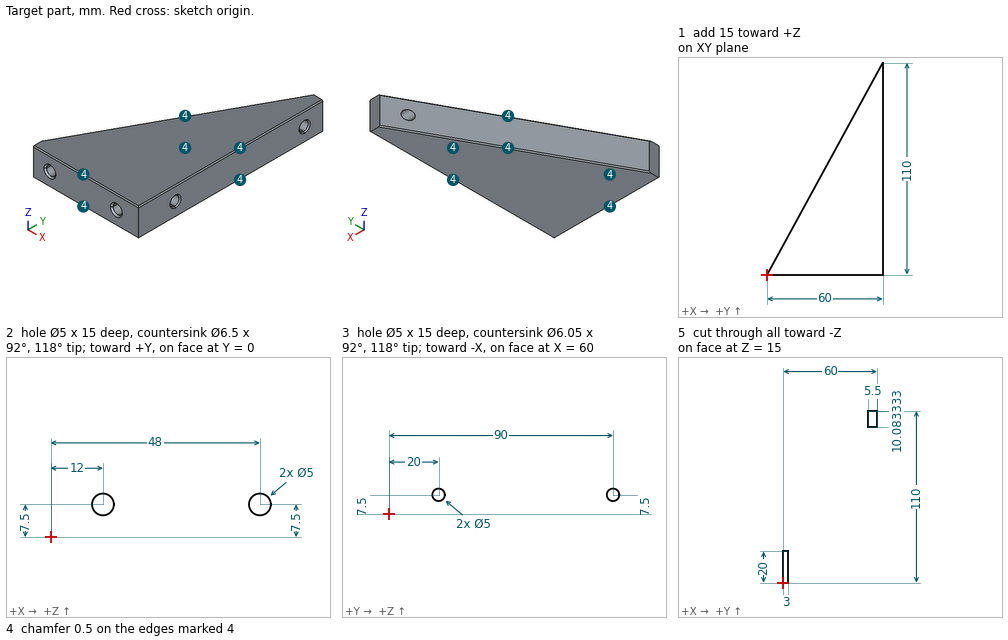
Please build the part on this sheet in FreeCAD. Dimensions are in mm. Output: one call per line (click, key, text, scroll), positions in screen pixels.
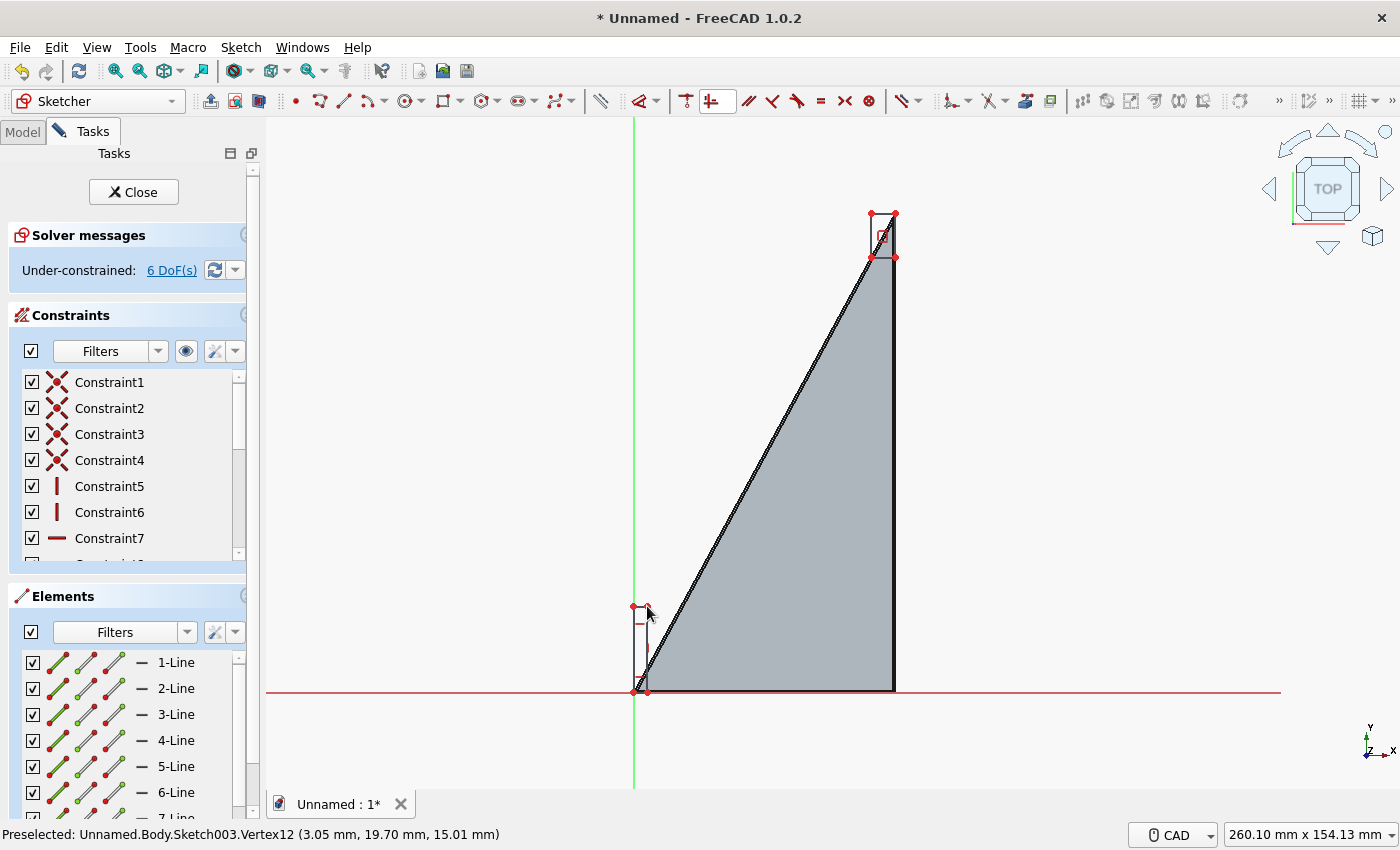
click(640, 102)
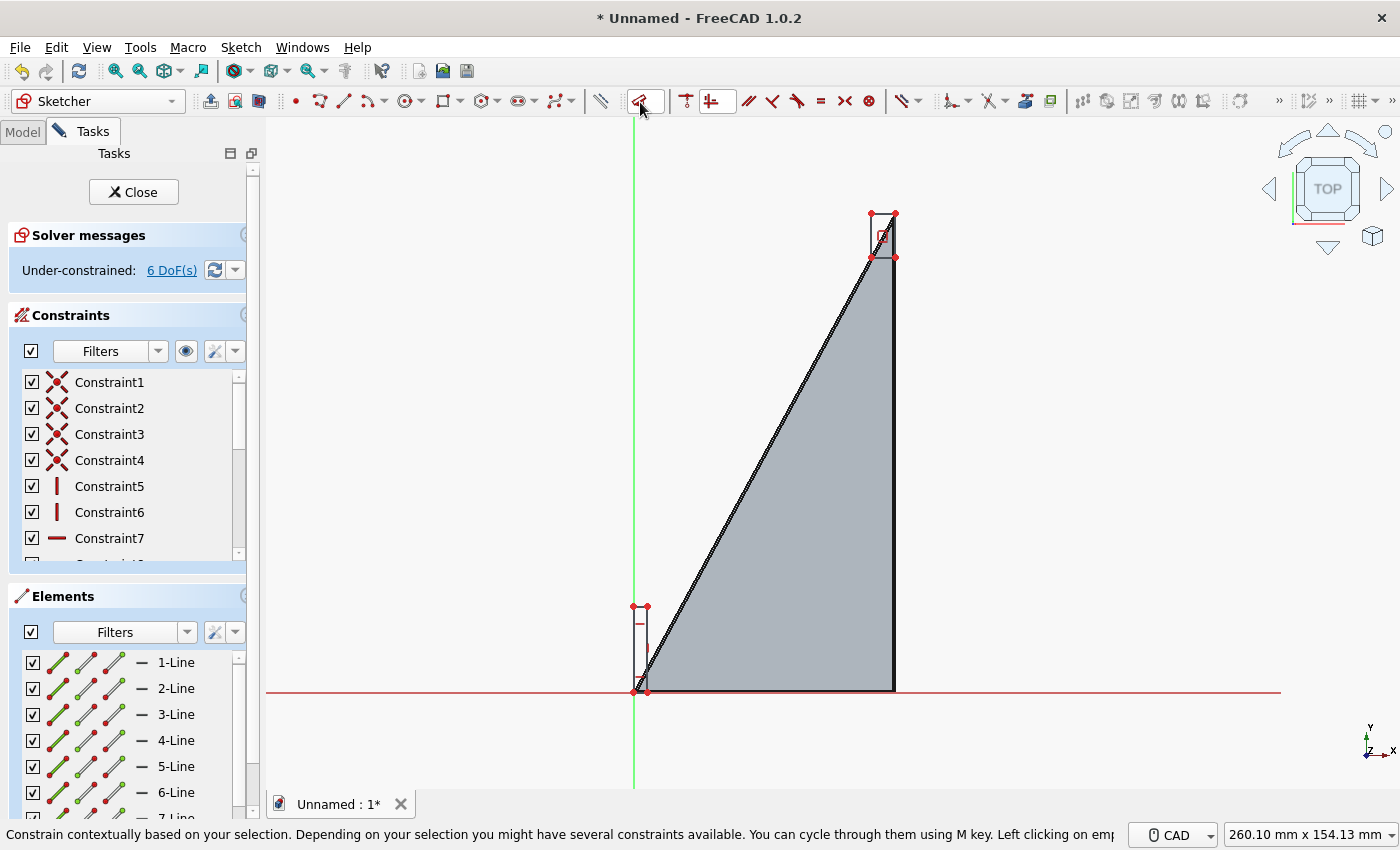
scroll(640, 693, up, 6)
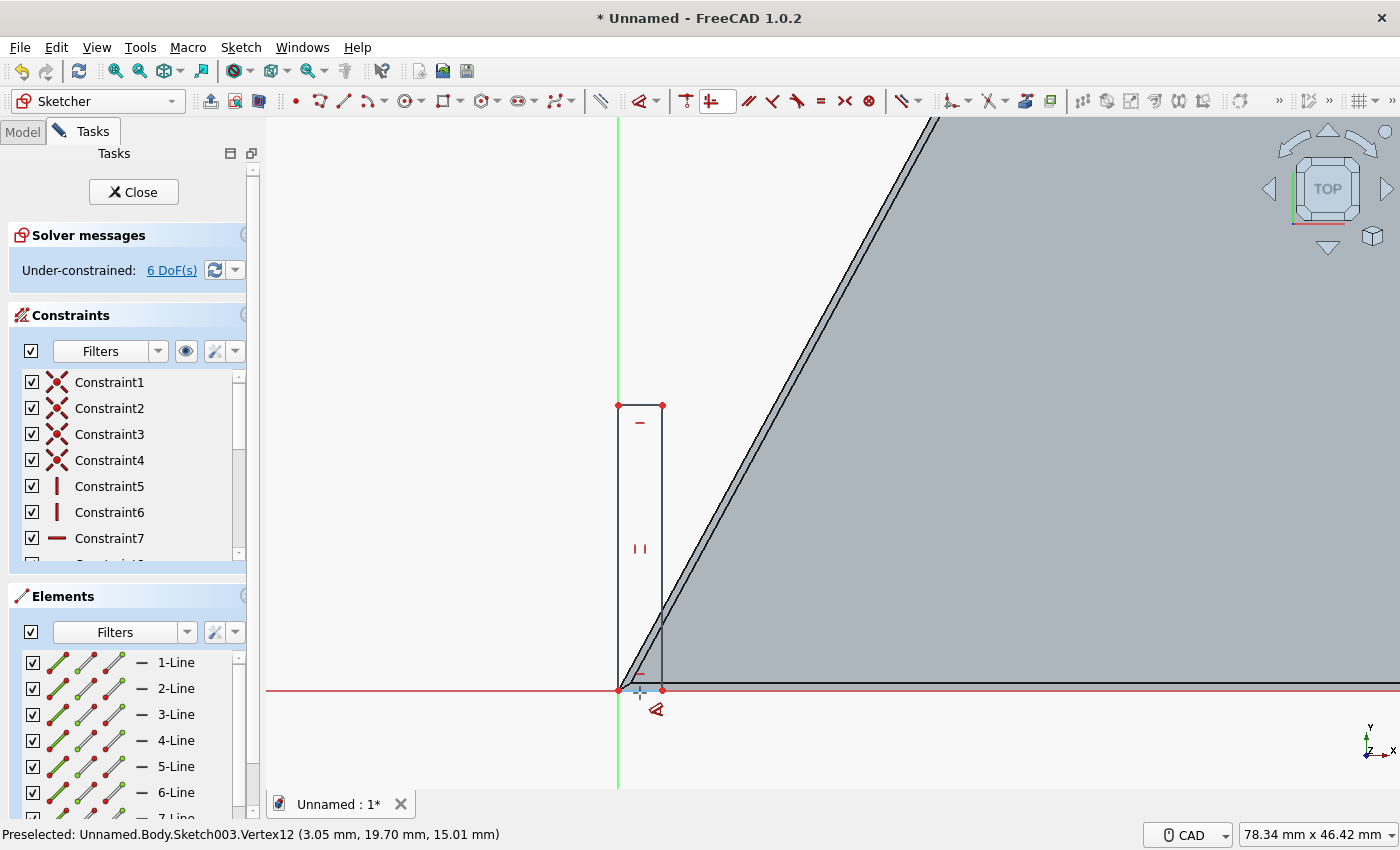
click(640, 691)
click(640, 725)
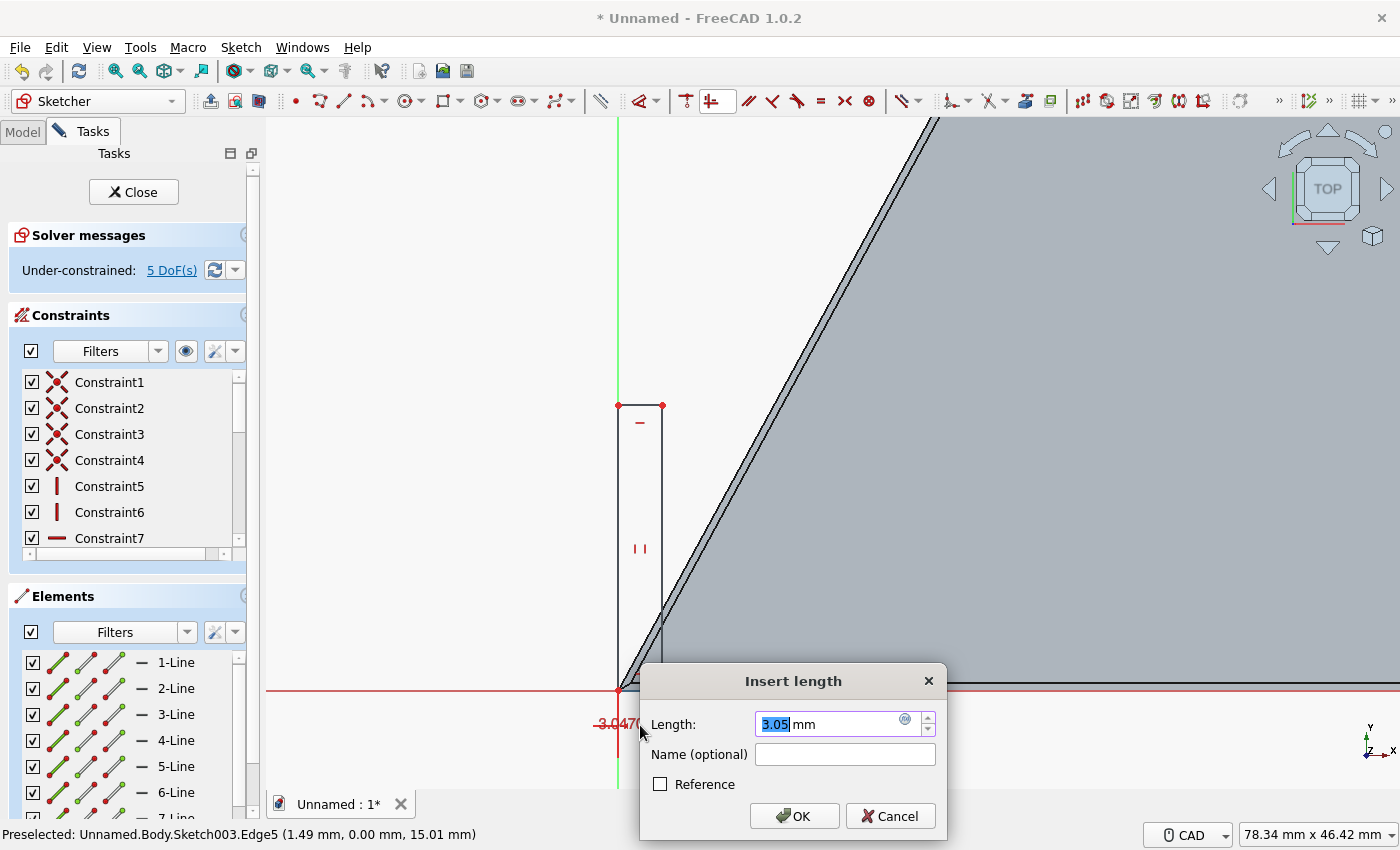
text(3)
key(Return)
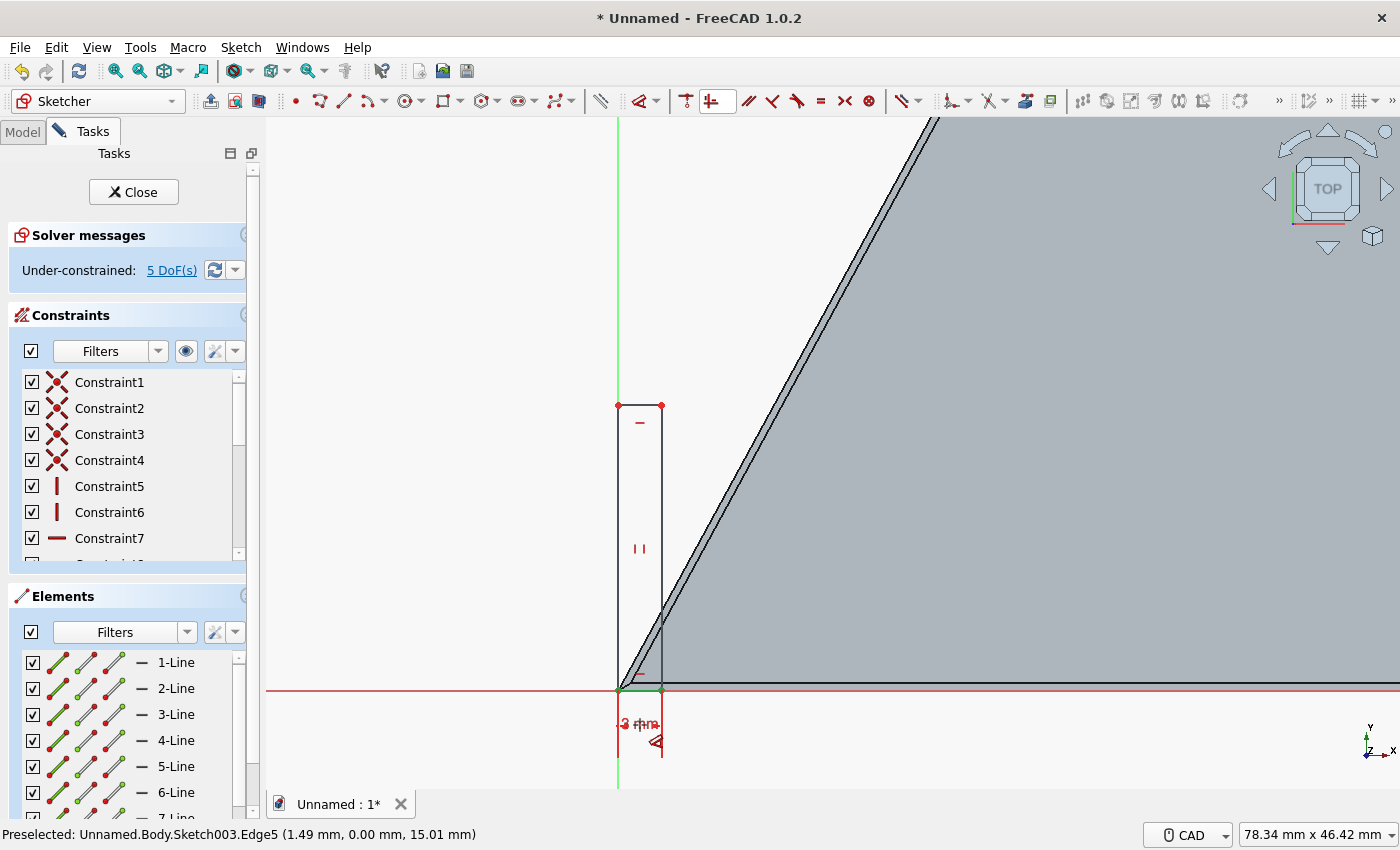
click(662, 605)
click(696, 548)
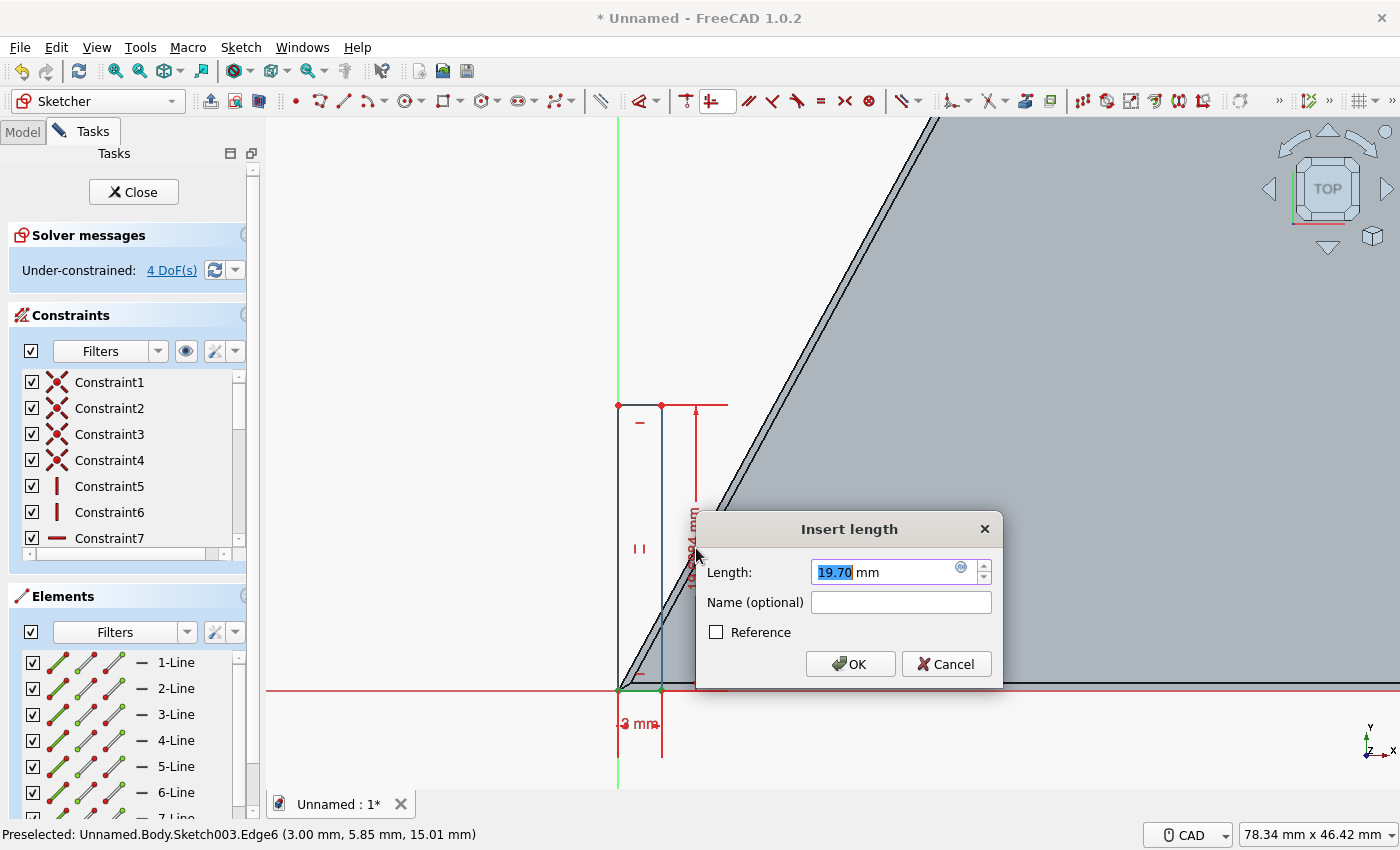
text(20)
key(Return)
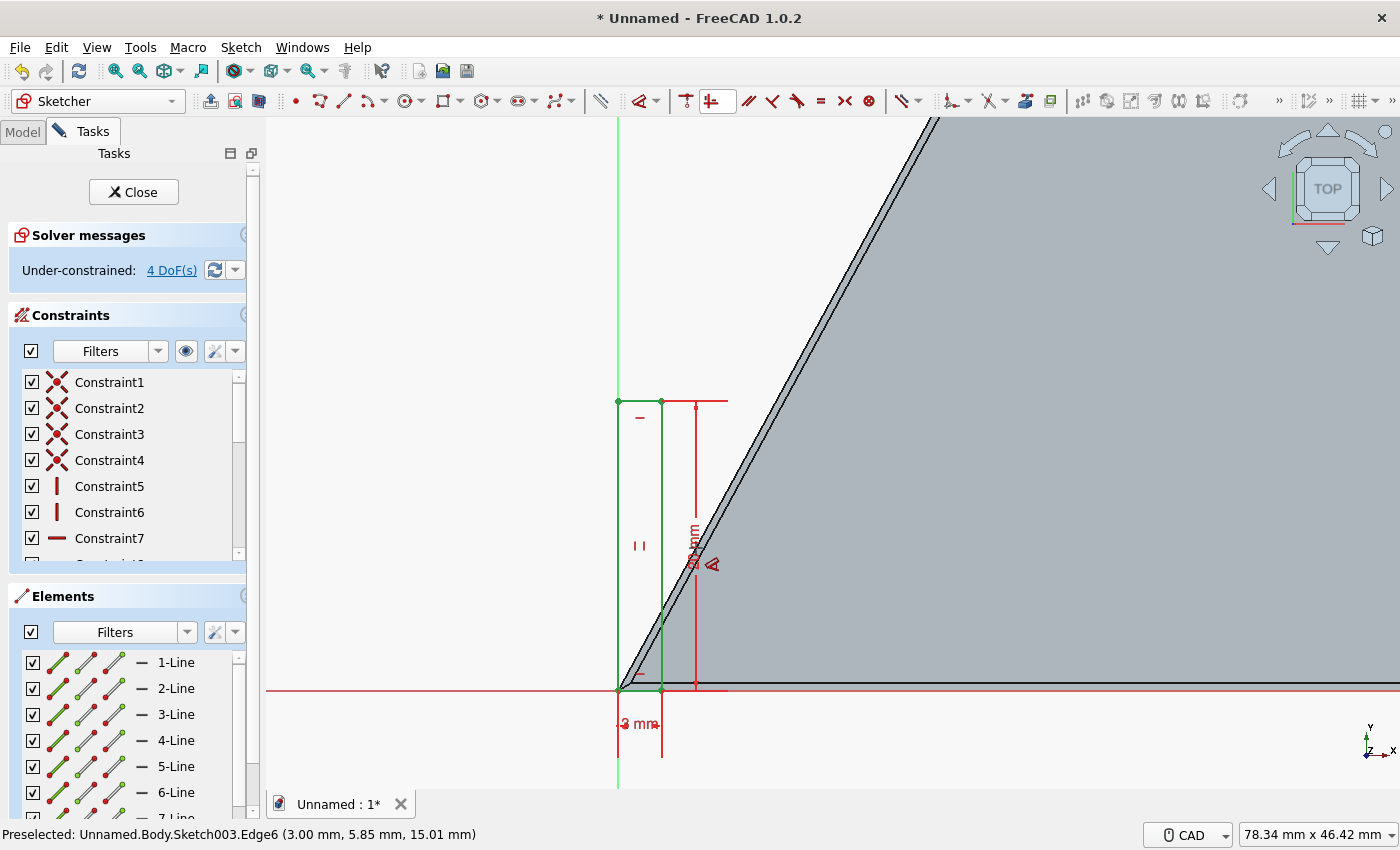
scroll(640, 694, down, 6)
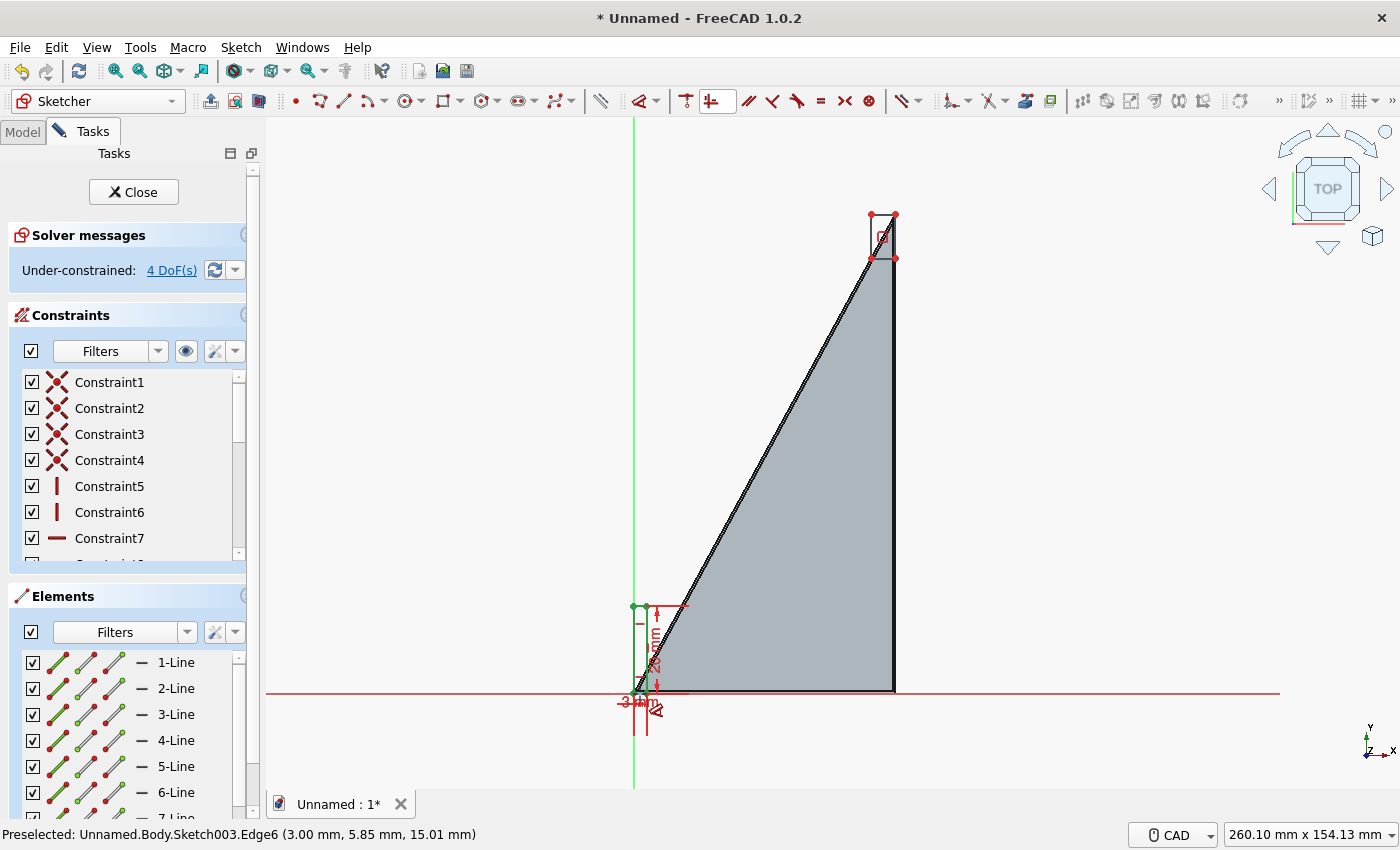
scroll(878, 259, up, 4)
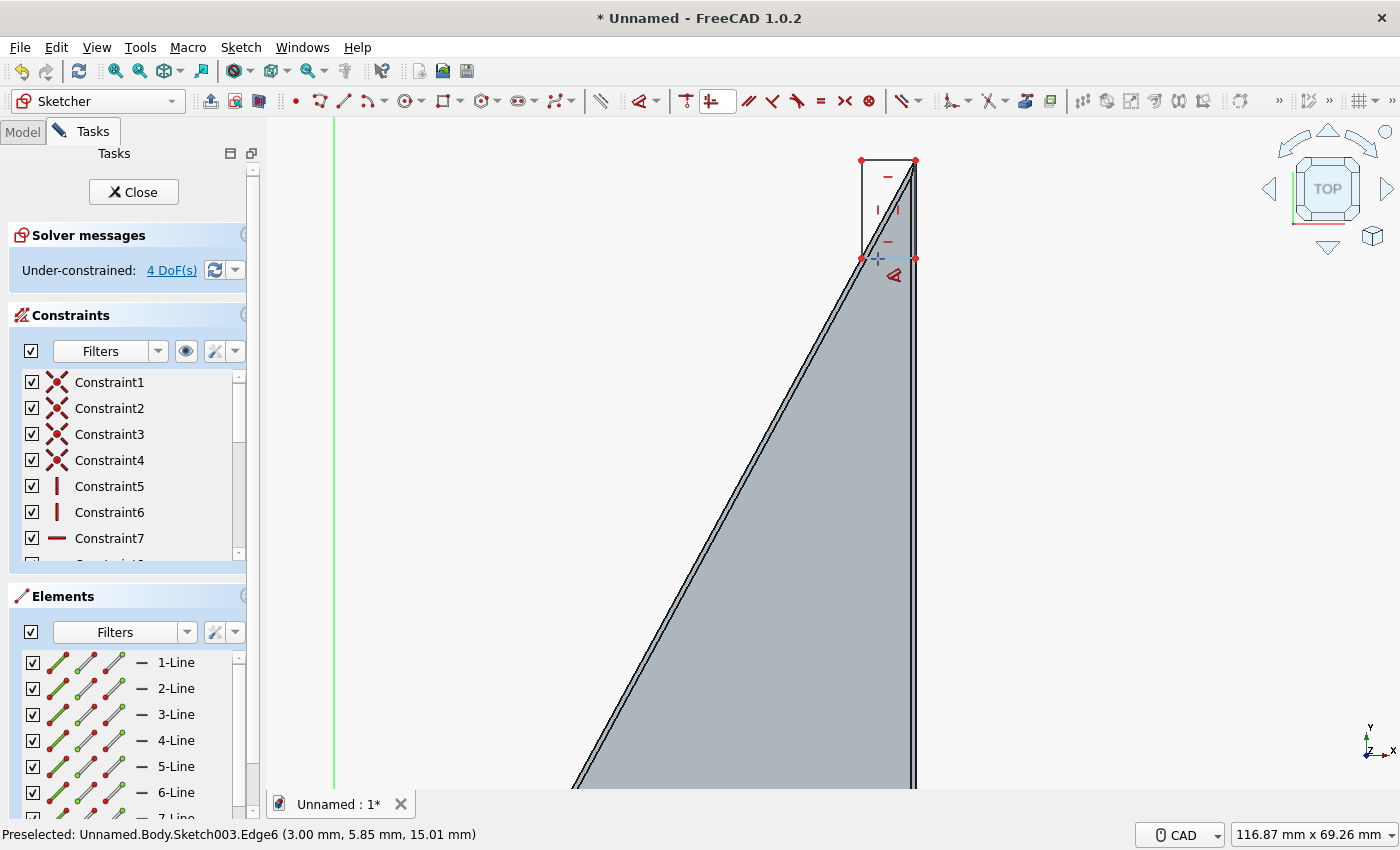
click(878, 258)
click(888, 224)